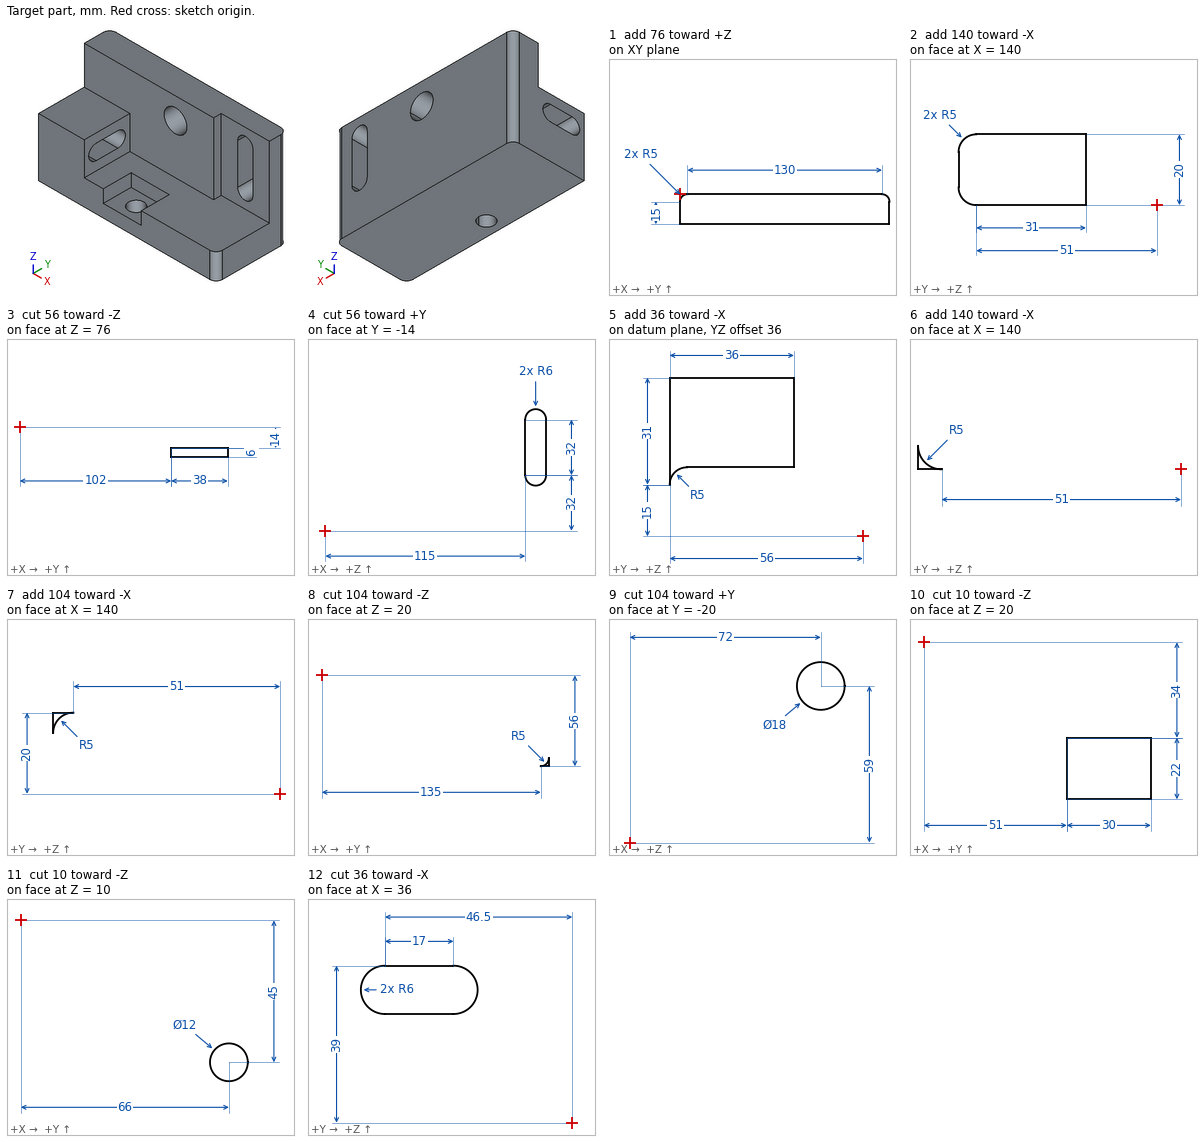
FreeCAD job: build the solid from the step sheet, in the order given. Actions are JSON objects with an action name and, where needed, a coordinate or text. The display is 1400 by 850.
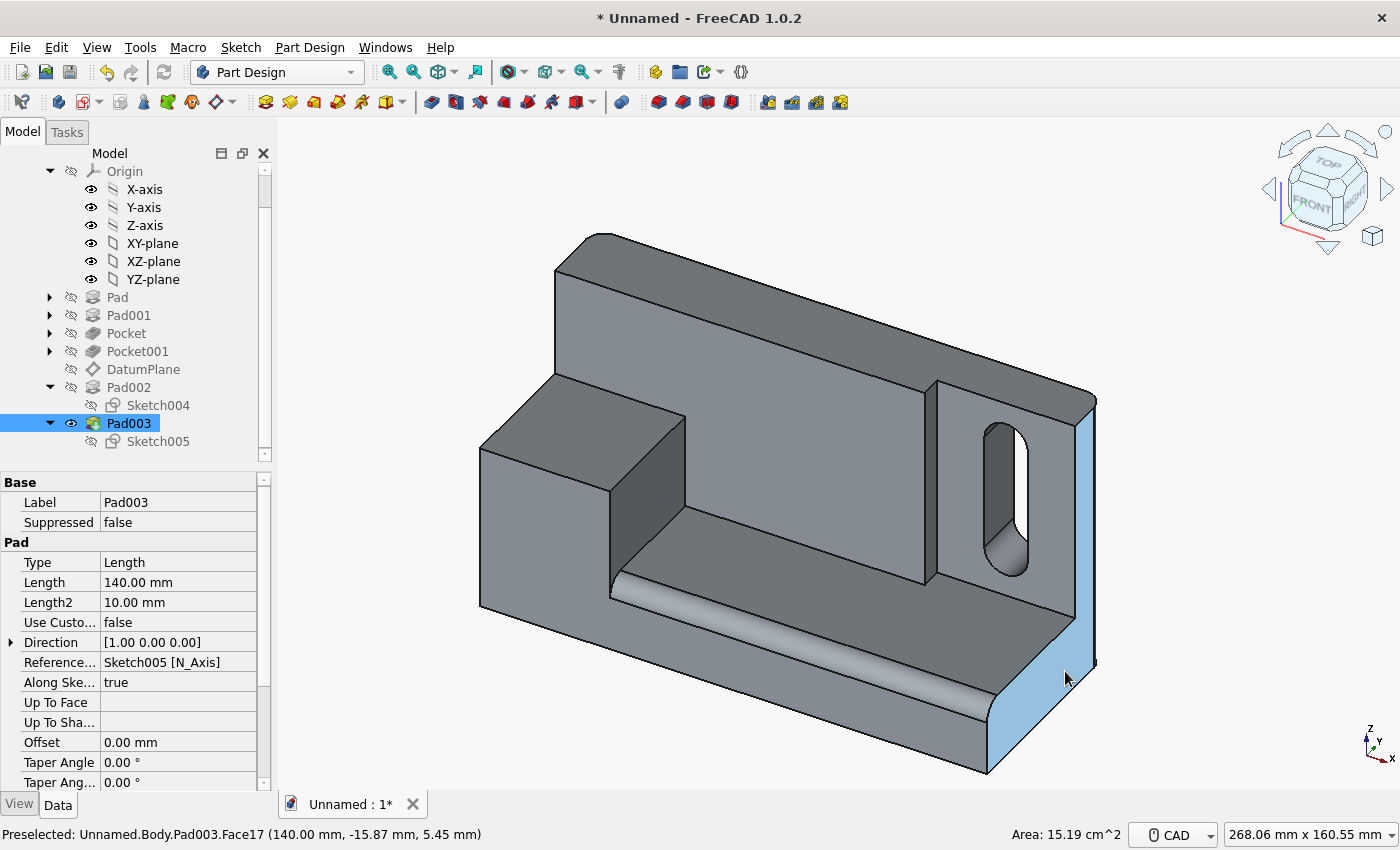
{"action": "left_click", "coordinate": [84, 102]}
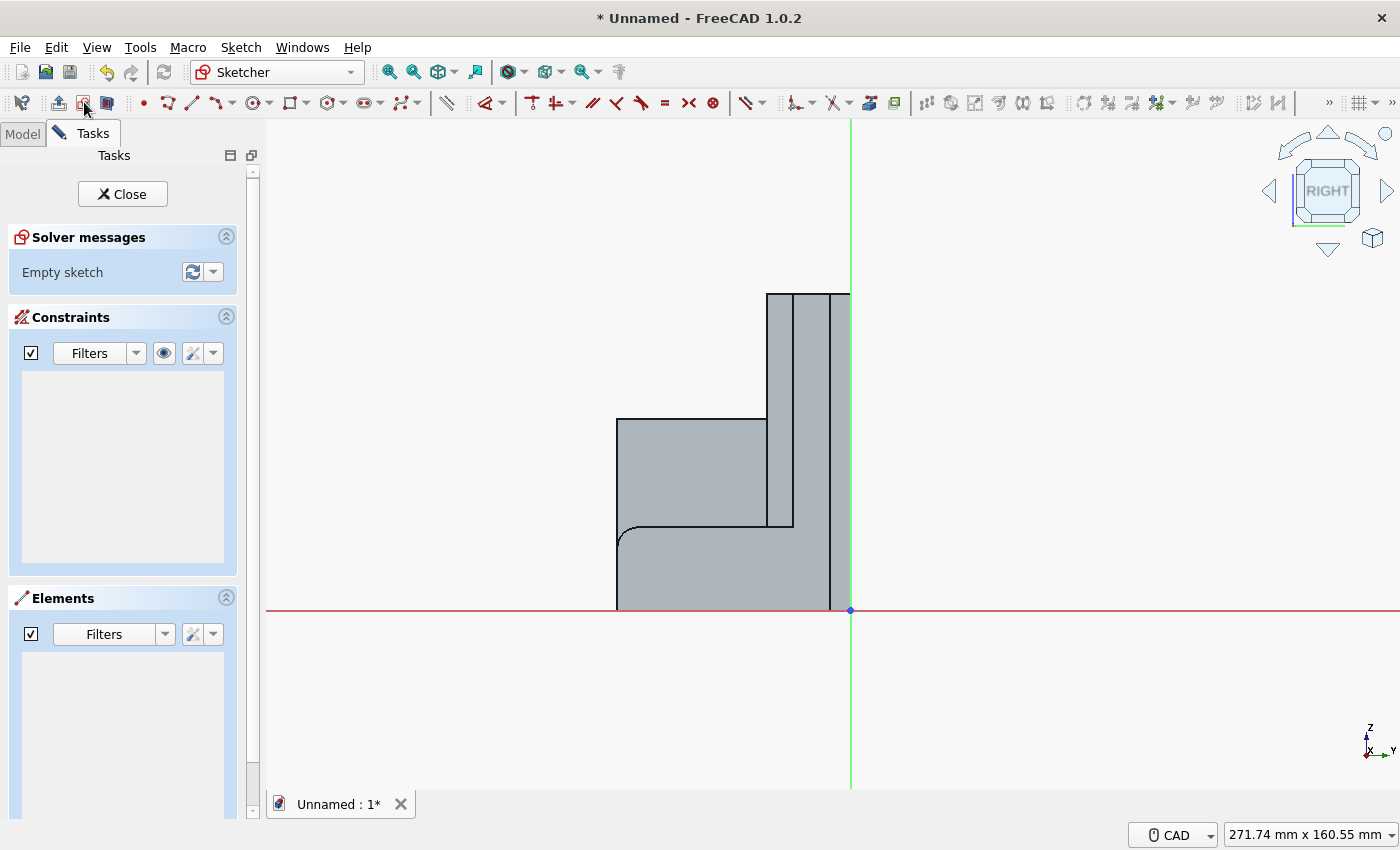
{"action": "scroll", "coordinate": [621, 542], "scroll_direction": "up", "scroll_amount": 15}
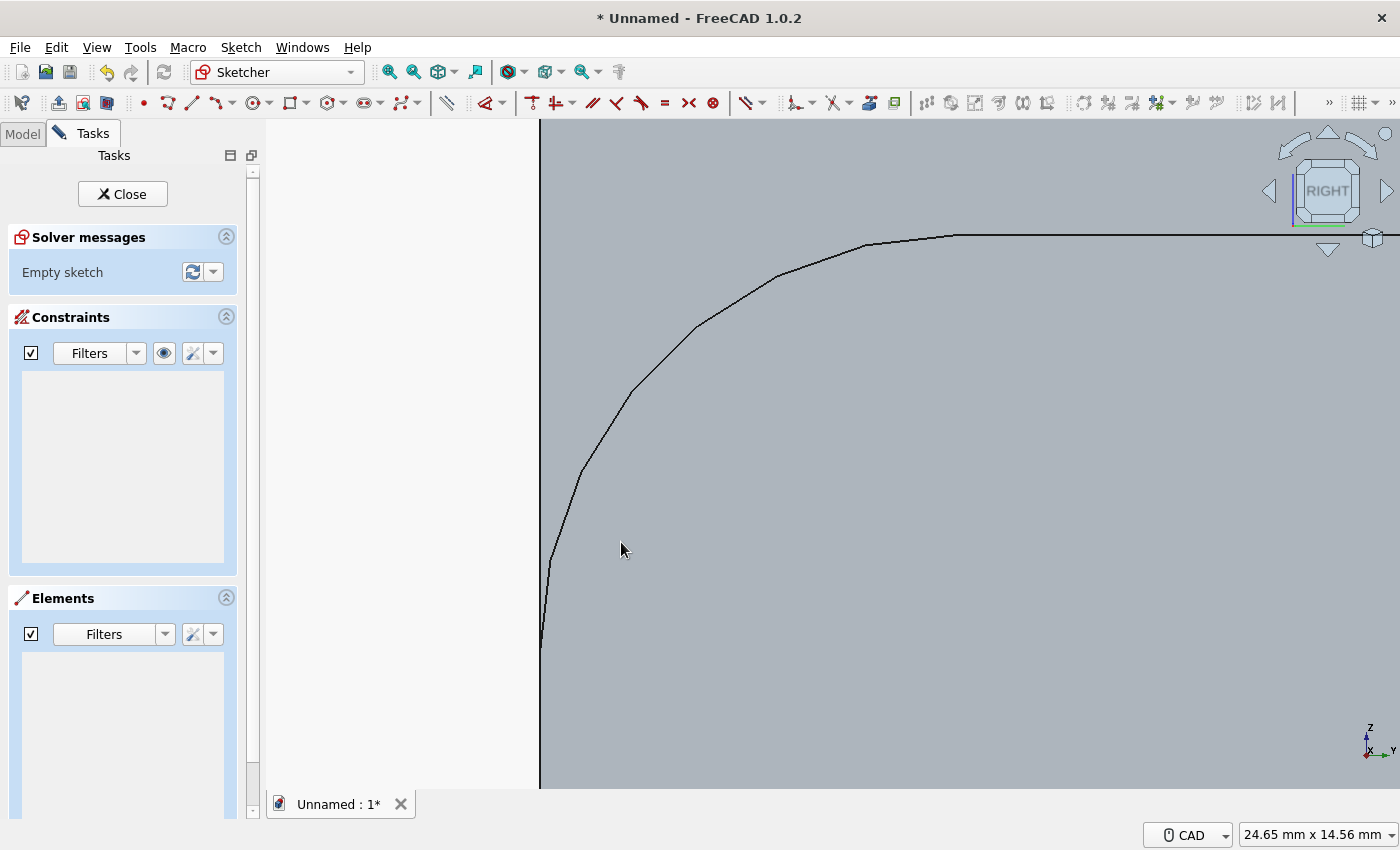
{"action": "left_click", "coordinate": [168, 104]}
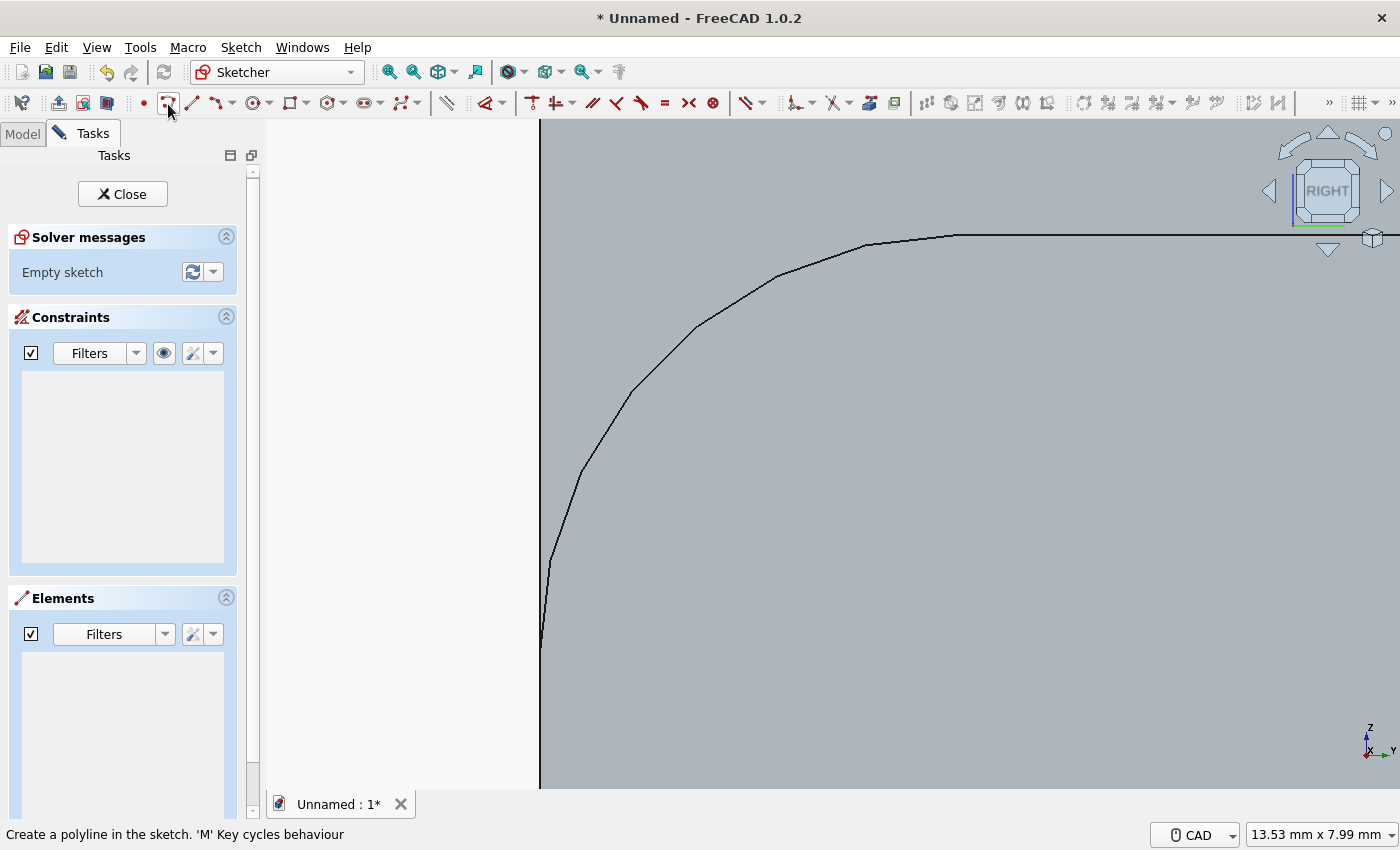
{"action": "left_click", "coordinate": [959, 235]}
{"action": "left_click", "coordinate": [540, 235]}
{"action": "left_click", "coordinate": [540, 654]}
{"action": "right_click", "coordinate": [540, 654]}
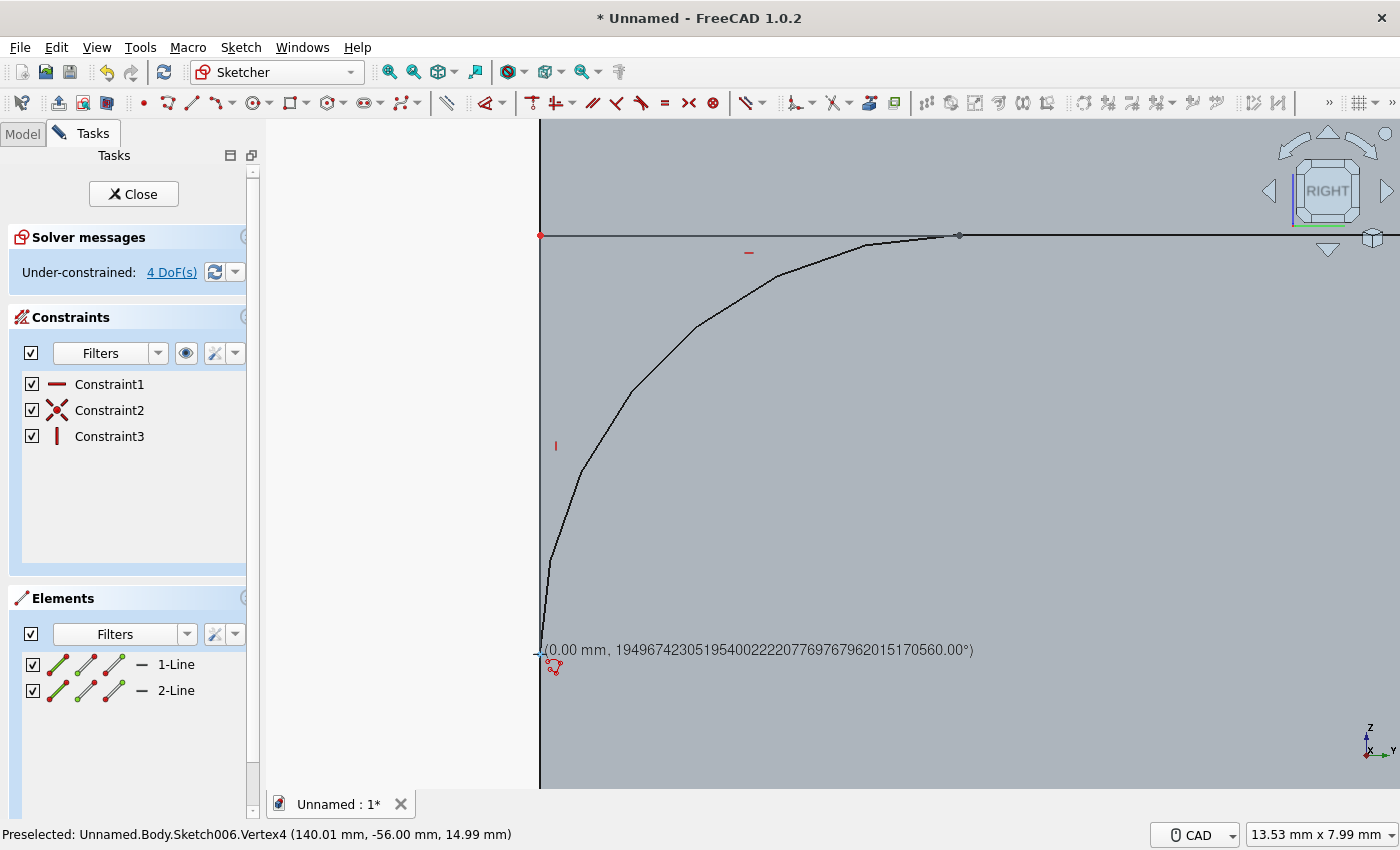
{"action": "key", "text": "g 3 a"}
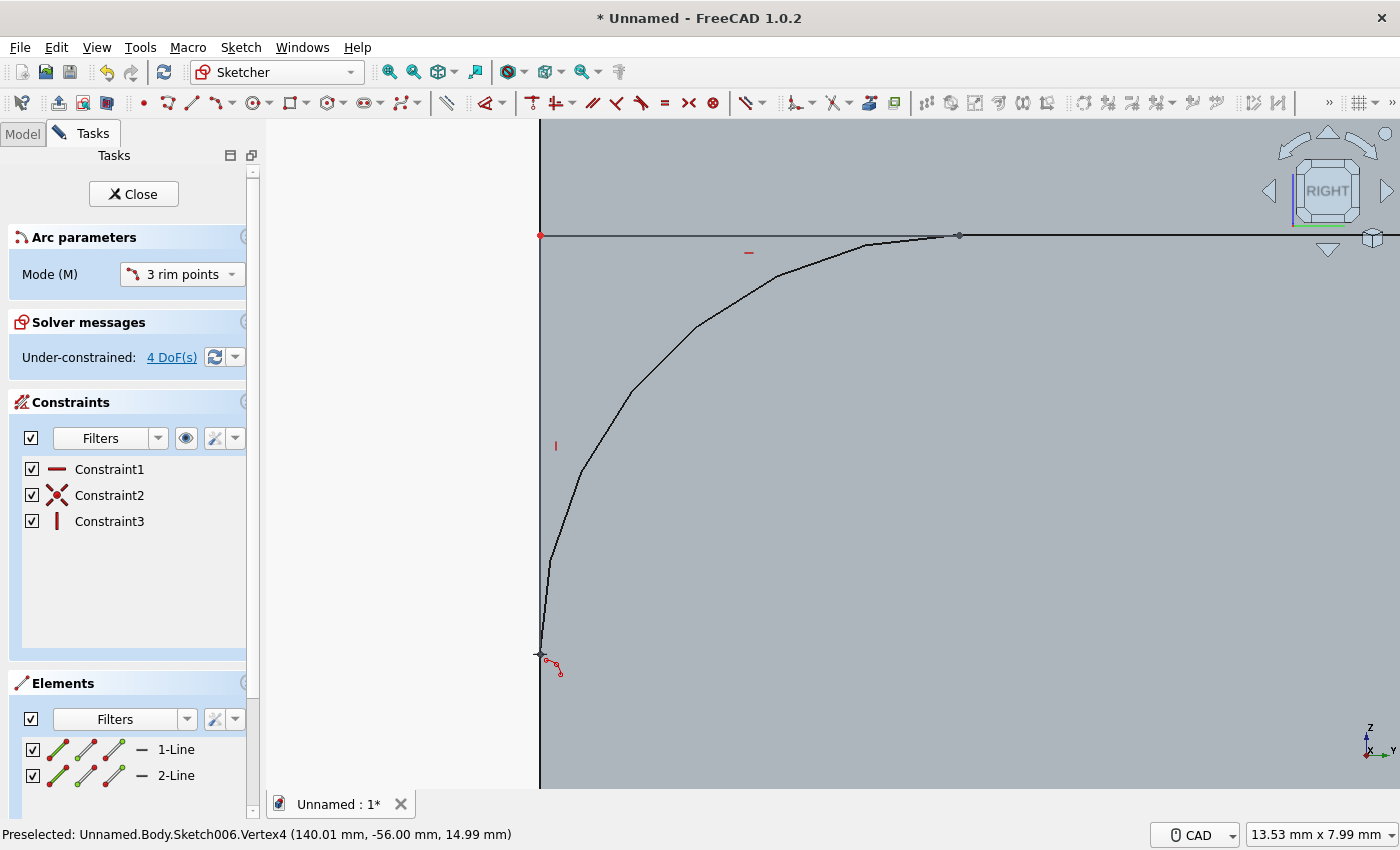
{"action": "left_click", "coordinate": [540, 655]}
{"action": "left_click", "coordinate": [959, 236]}
{"action": "left_click", "coordinate": [663, 358]}
{"action": "key", "text": "Escape"}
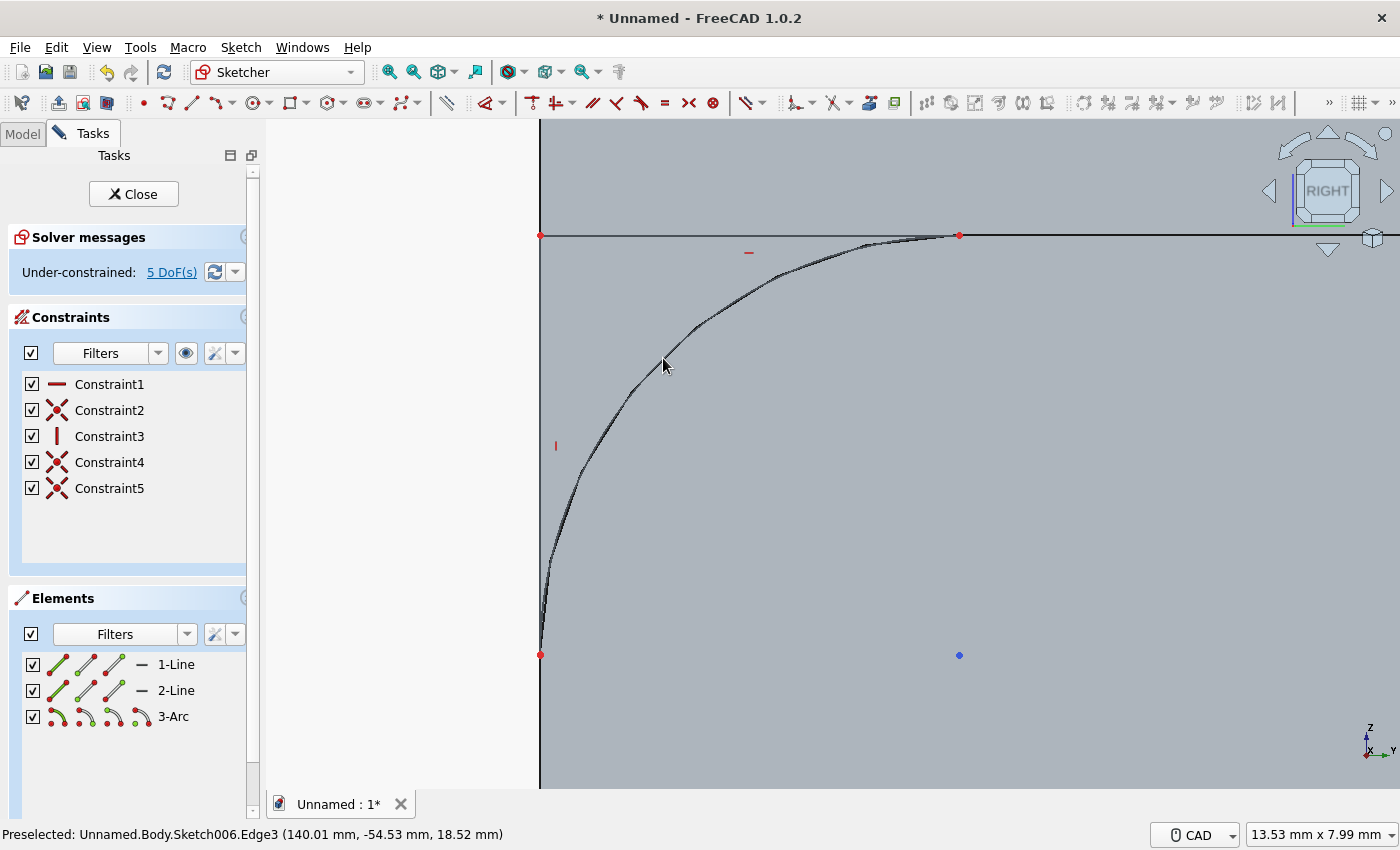
{"action": "left_click", "coordinate": [833, 236]}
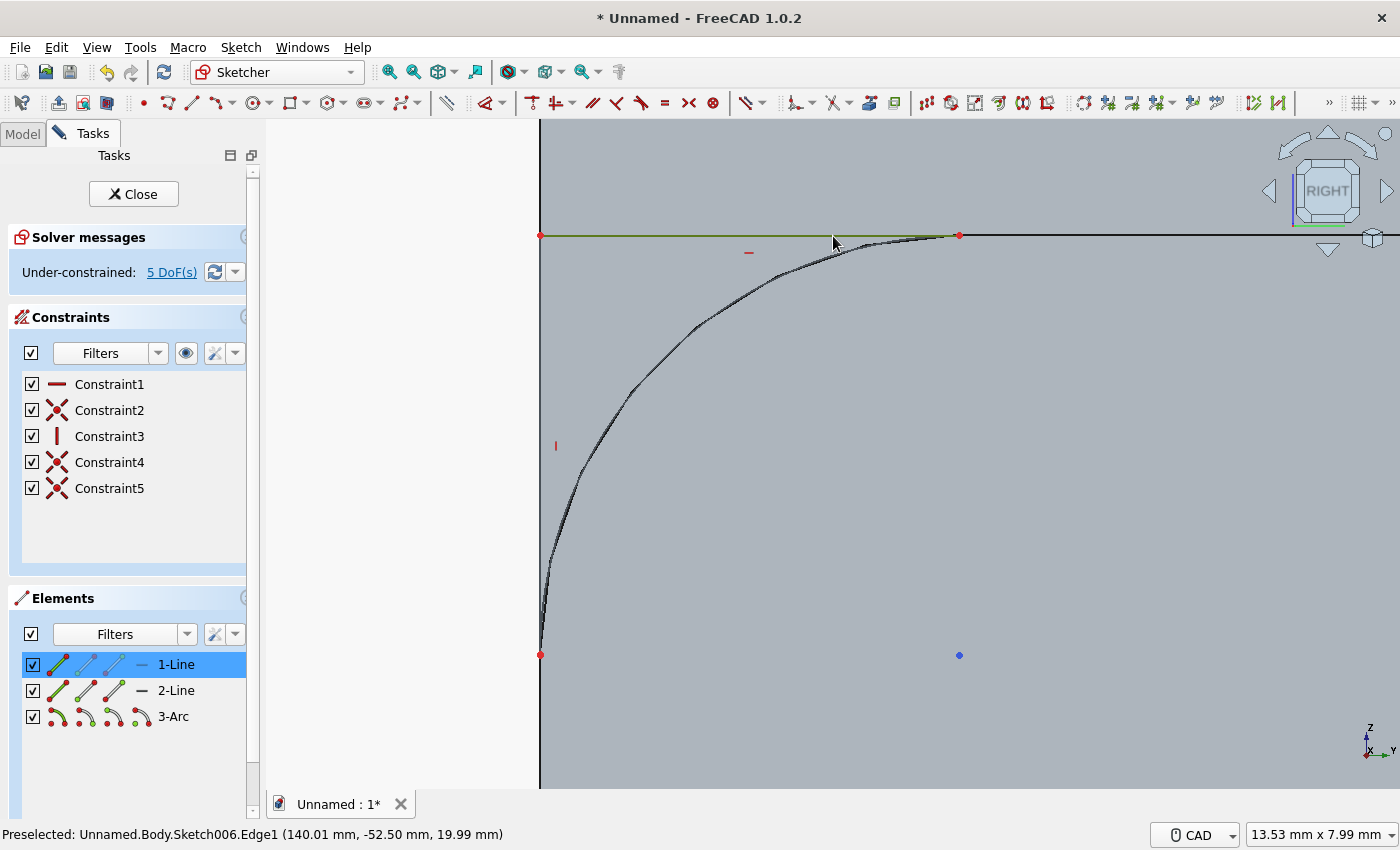
{"action": "left_click", "coordinate": [769, 282]}